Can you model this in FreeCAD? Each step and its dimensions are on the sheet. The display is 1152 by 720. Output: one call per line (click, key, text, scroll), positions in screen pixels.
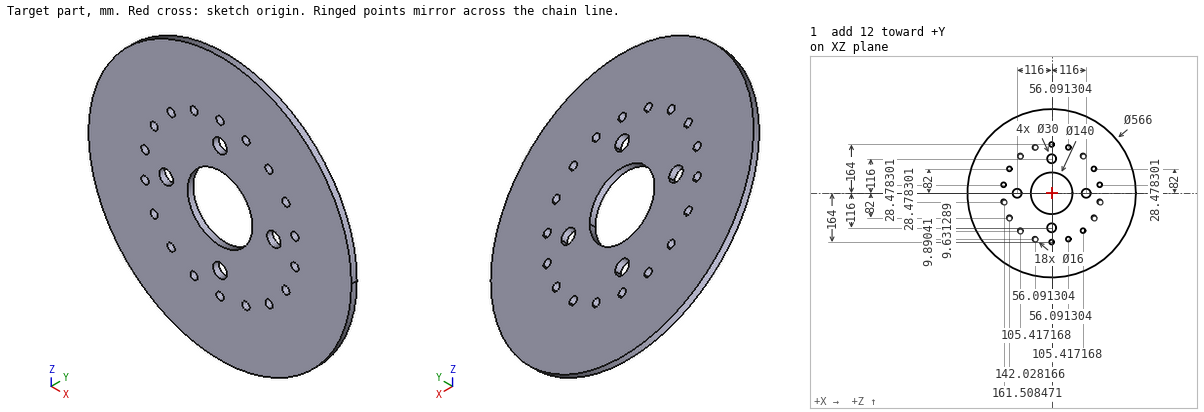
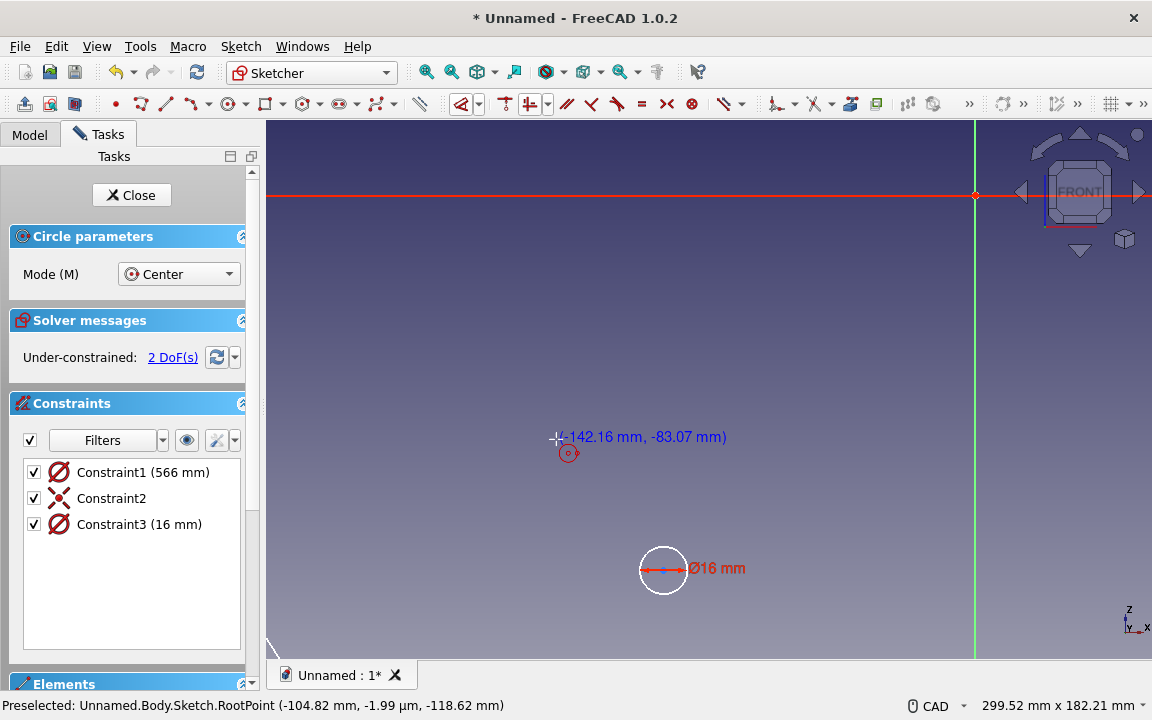
scroll(556, 438, down, 8)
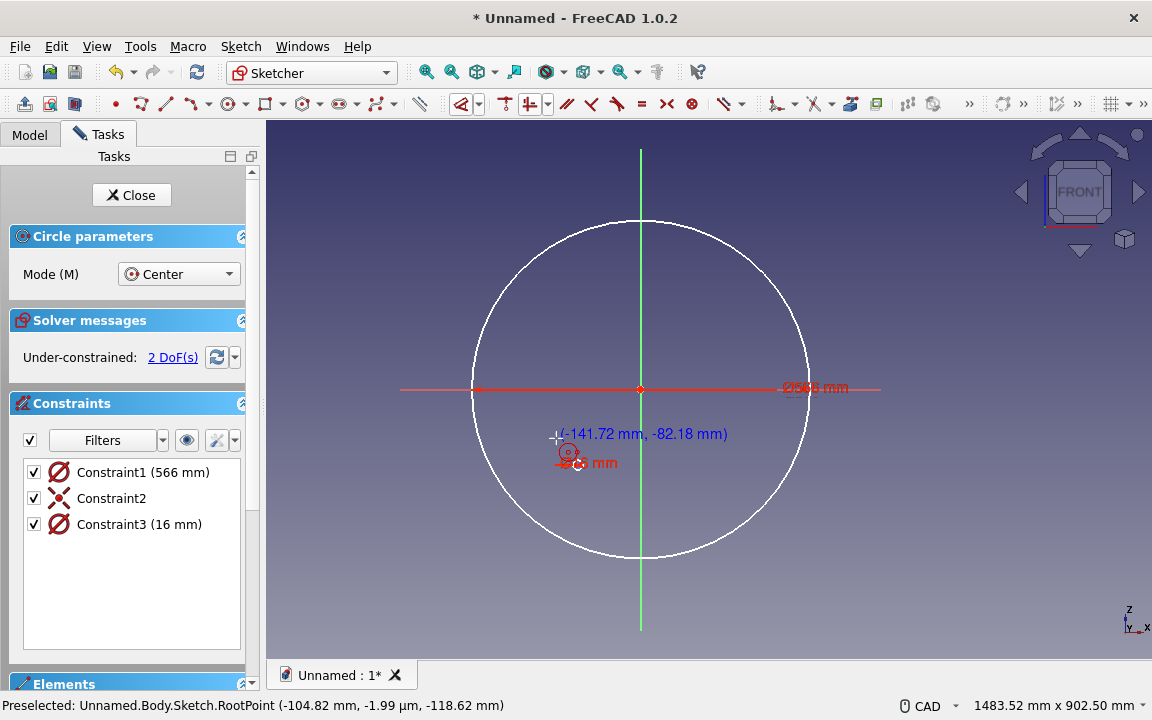
click(556, 439)
move(559, 435)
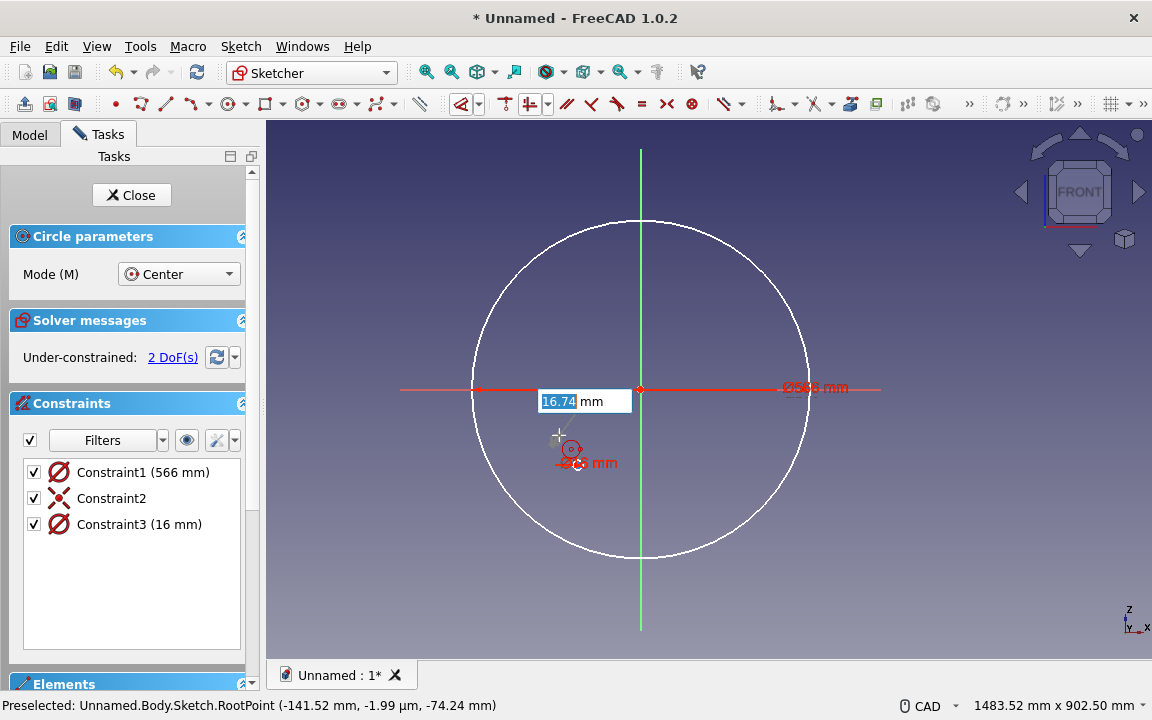
text(16)
key(Return)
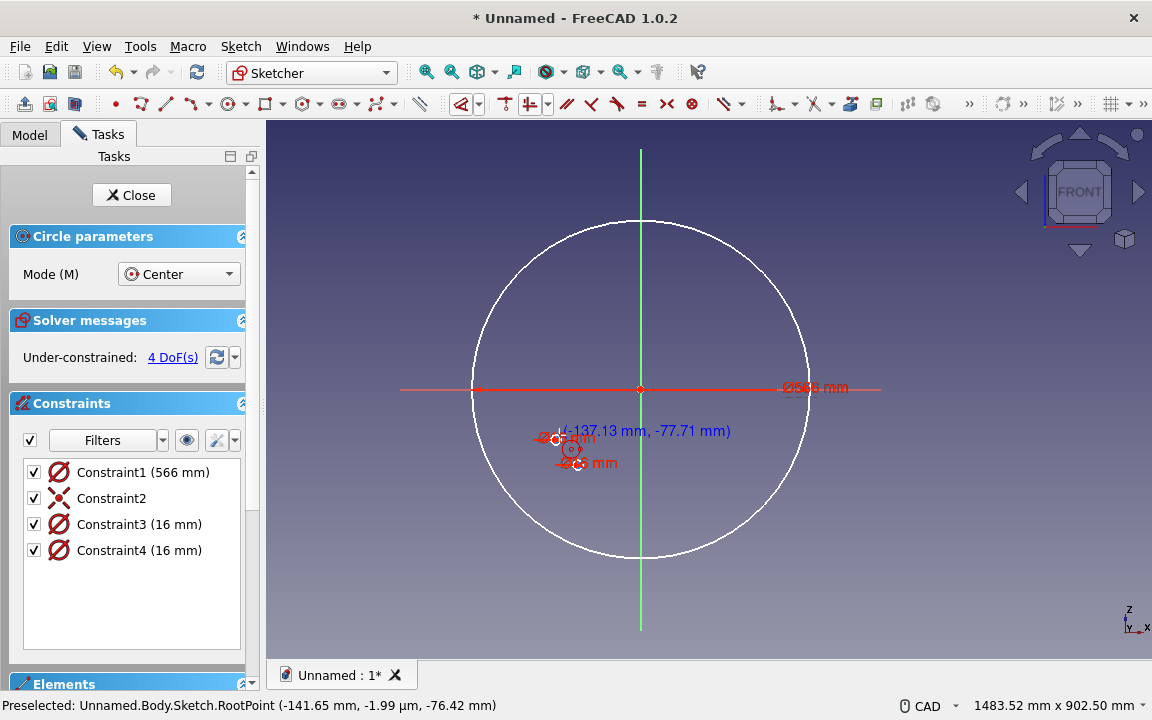
scroll(544, 407, up, 8)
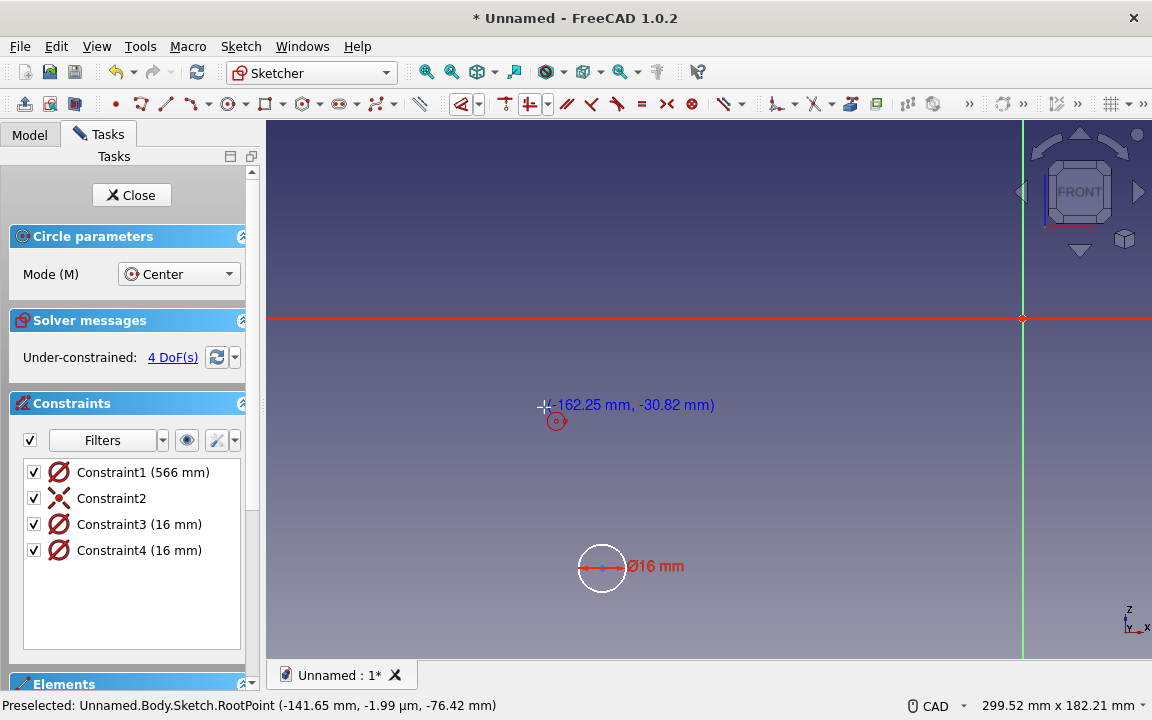
scroll(544, 407, down, 8)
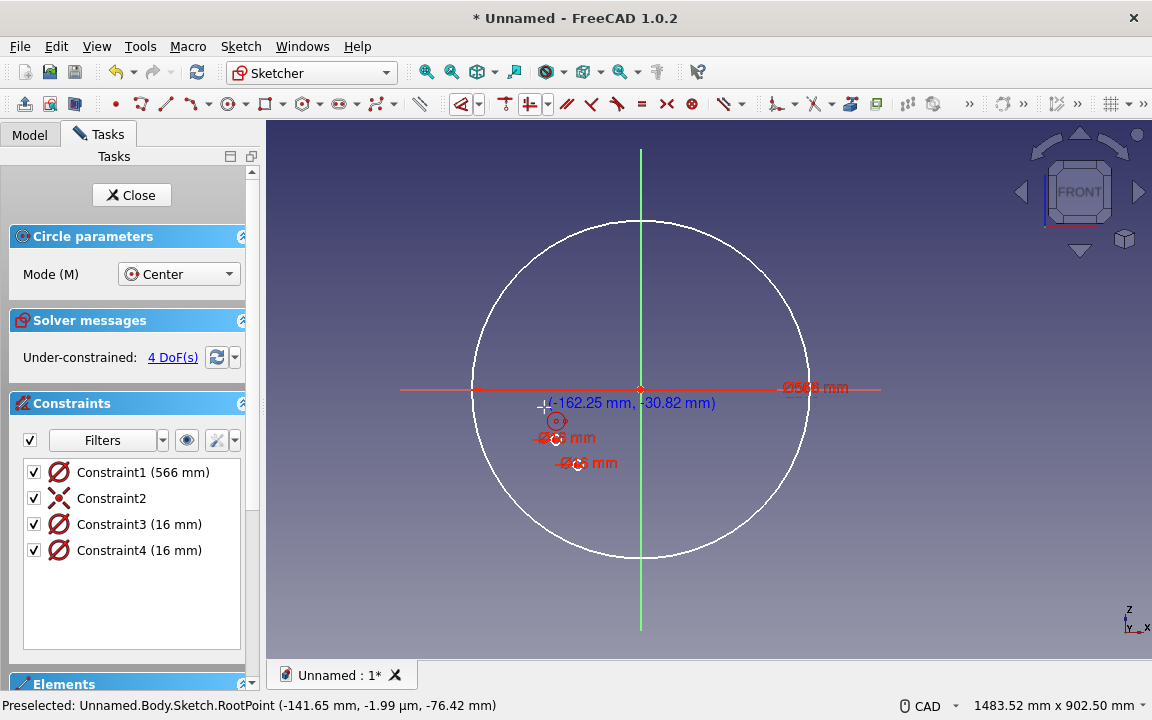
click(544, 407)
move(548, 410)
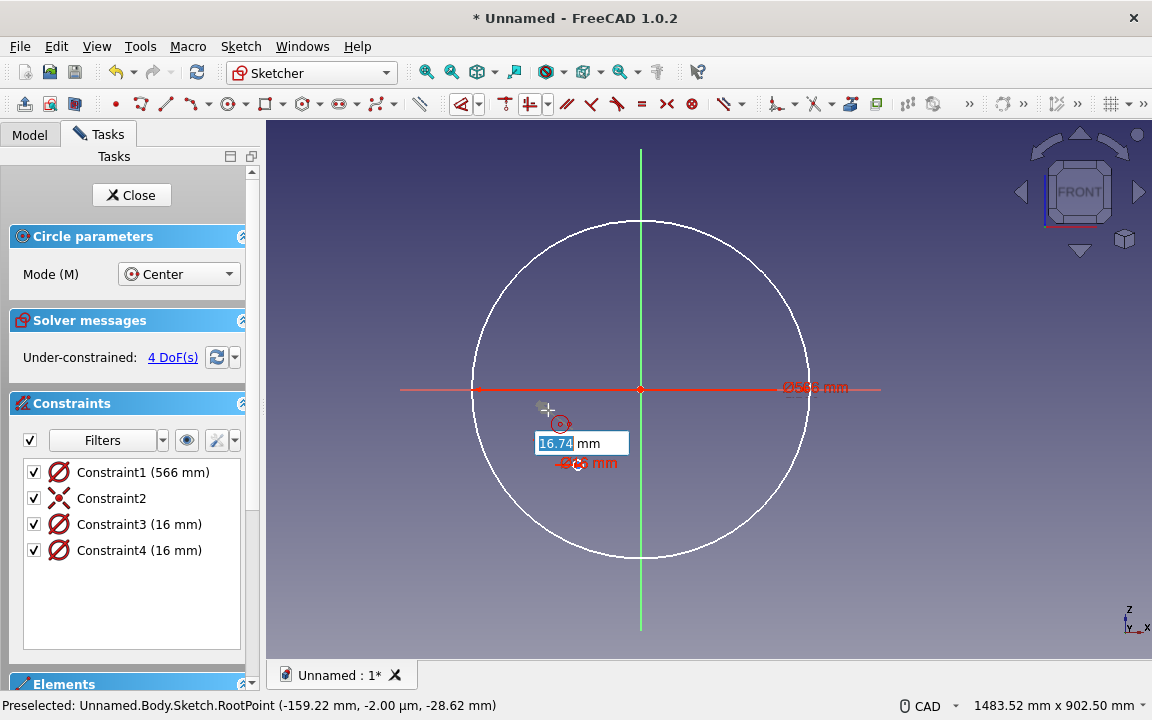
text(16)
key(Return)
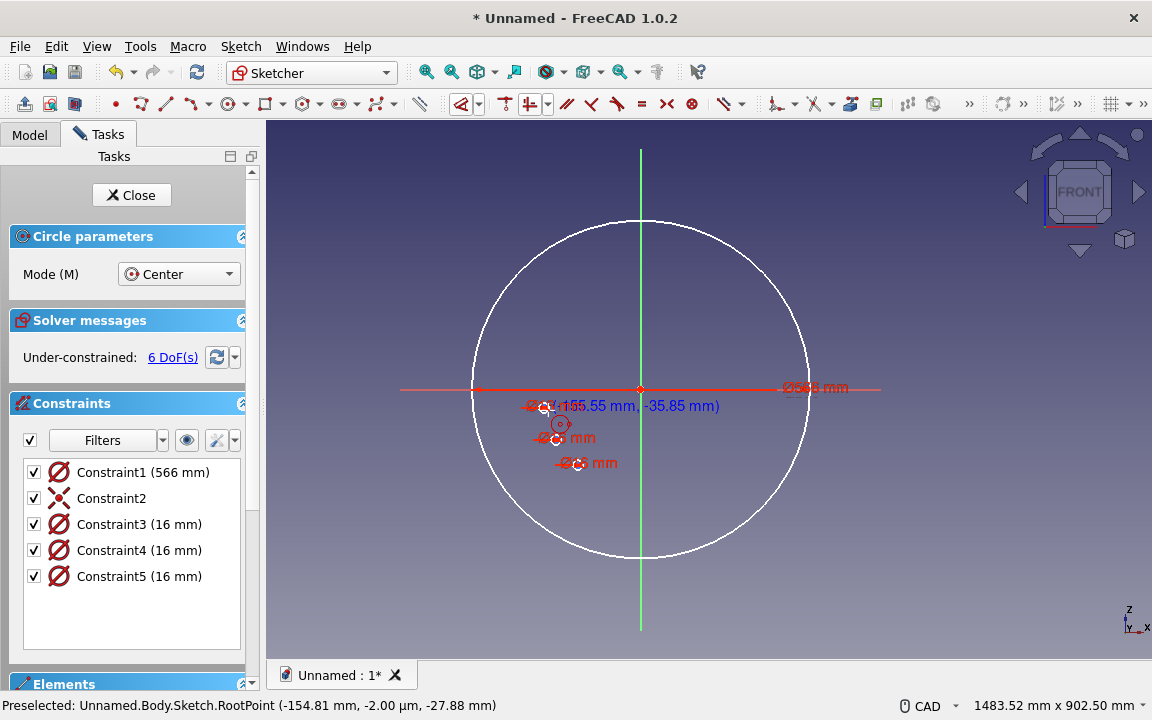
scroll(607, 482, up, 8)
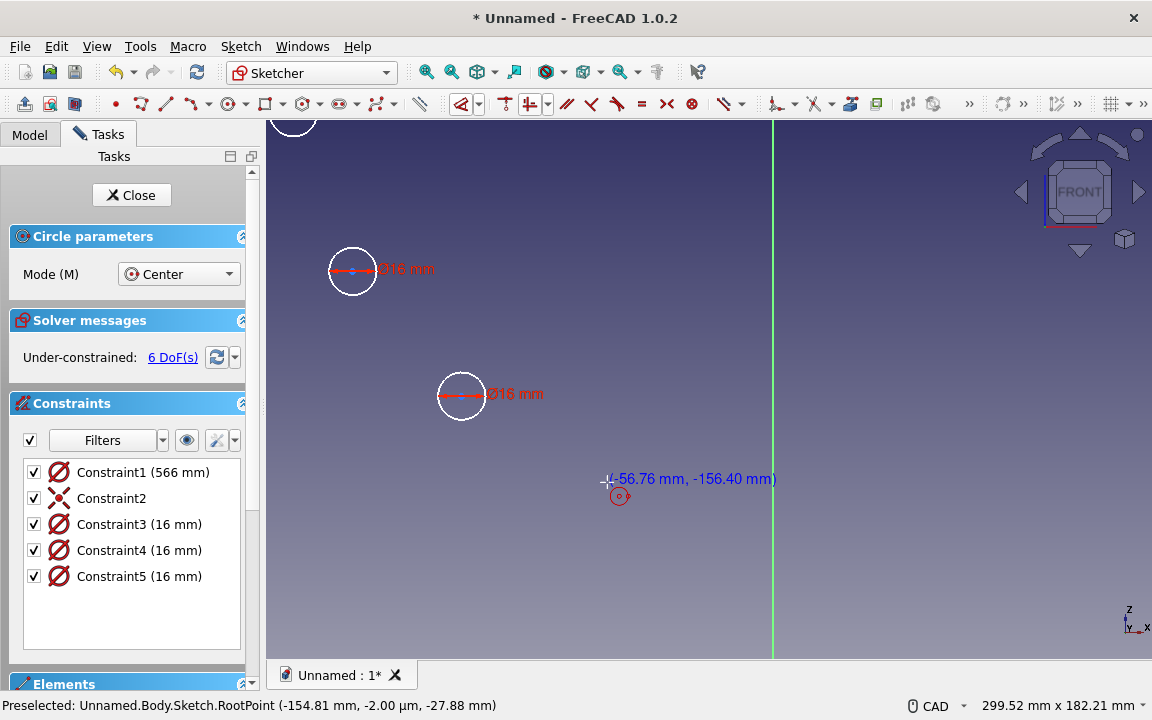
scroll(607, 483, down, 8)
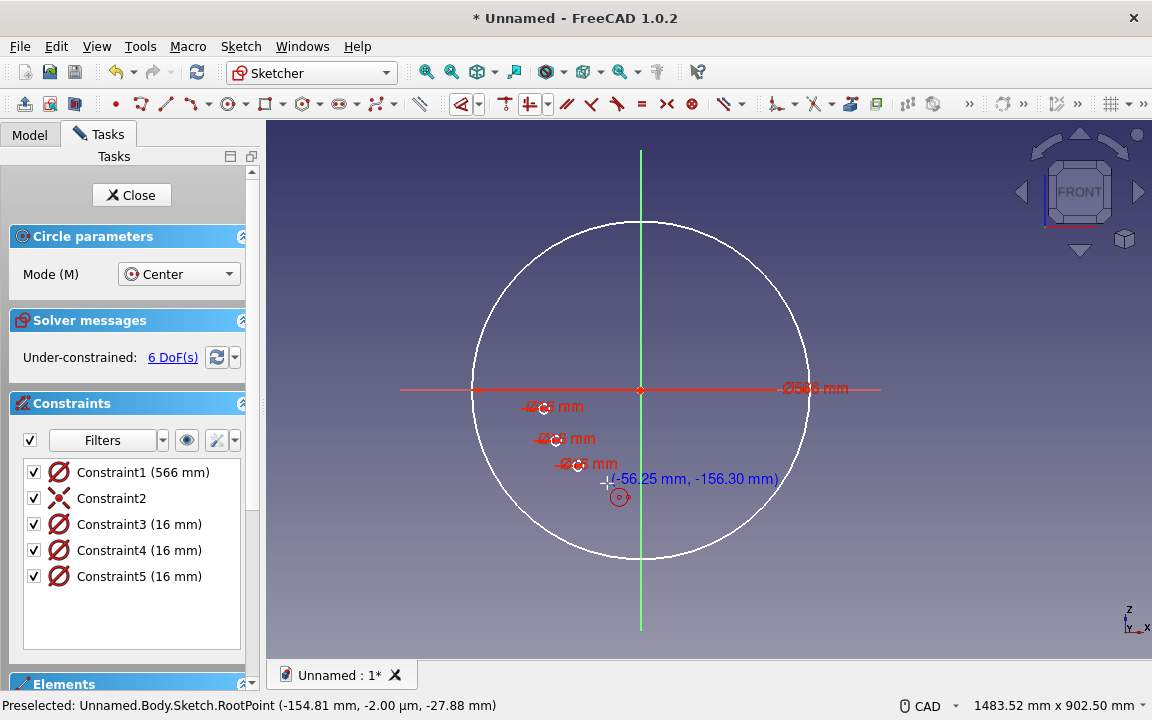
click(607, 482)
move(611, 479)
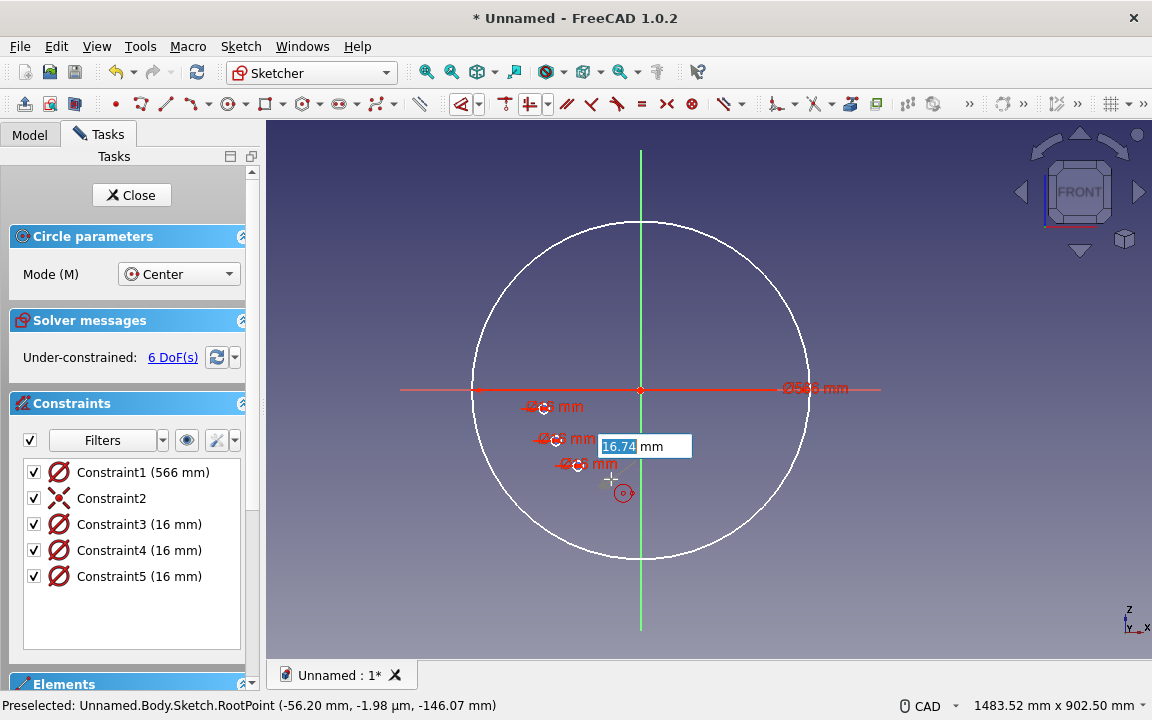
text(16)
key(Return)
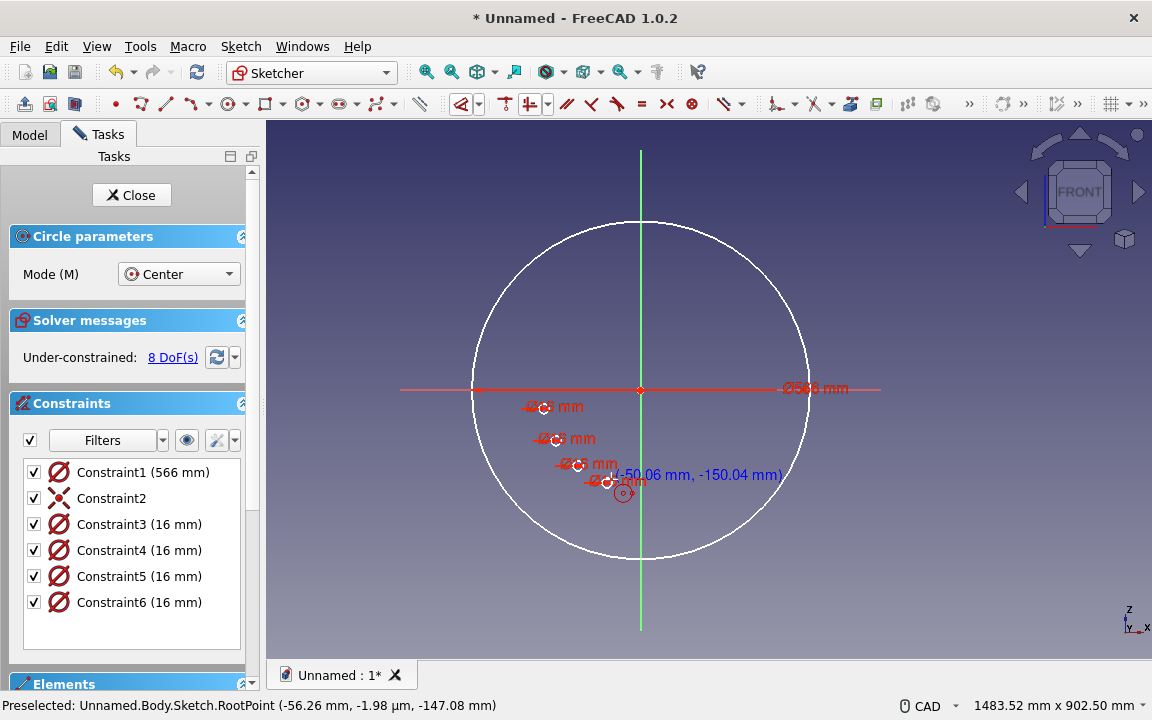
scroll(641, 488, up, 8)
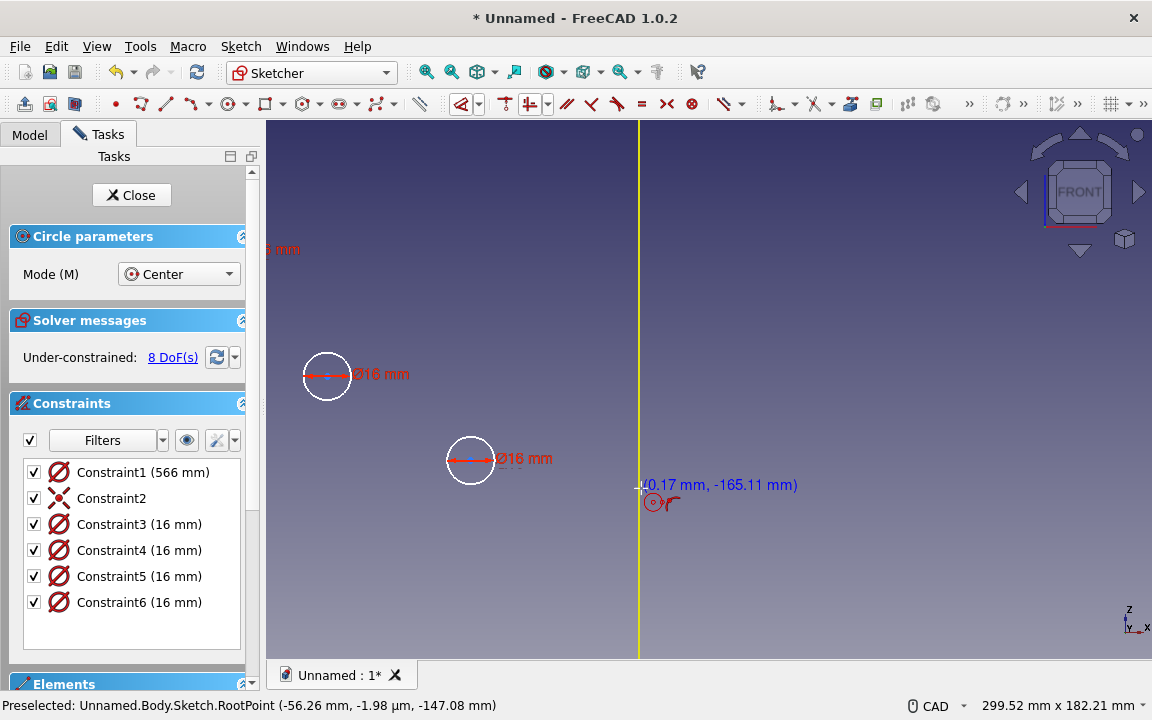
scroll(641, 488, down, 8)